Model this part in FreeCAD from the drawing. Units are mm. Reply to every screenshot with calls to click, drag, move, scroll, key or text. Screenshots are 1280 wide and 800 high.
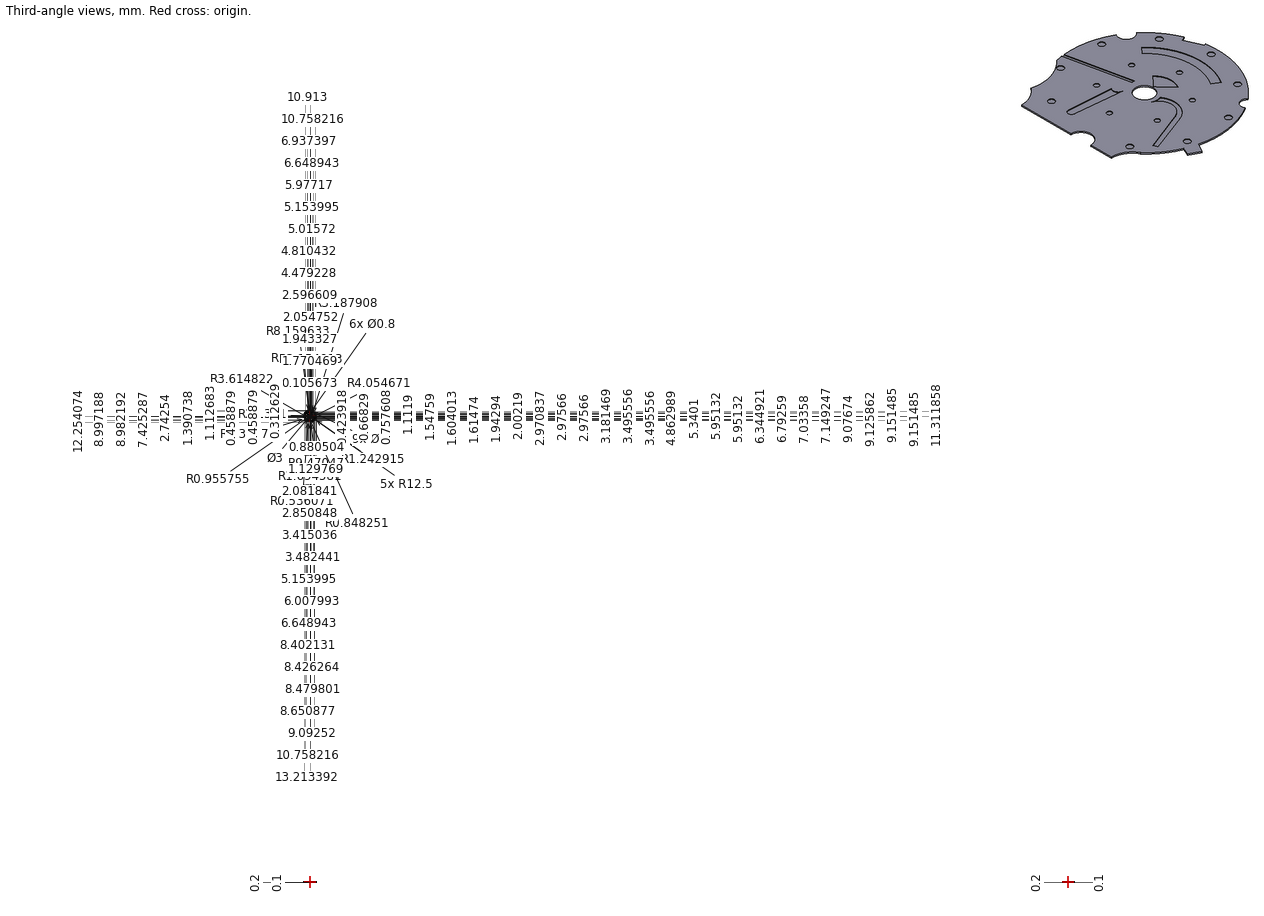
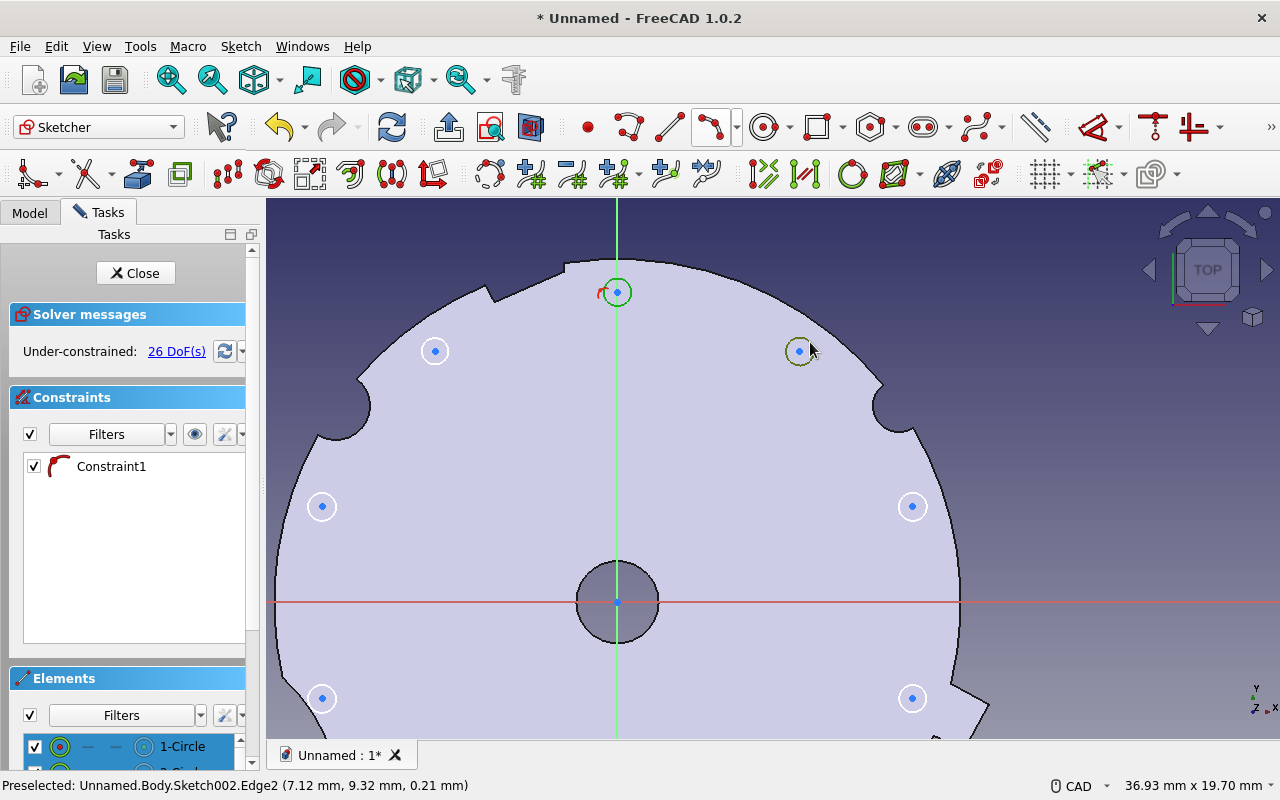
click(923, 497)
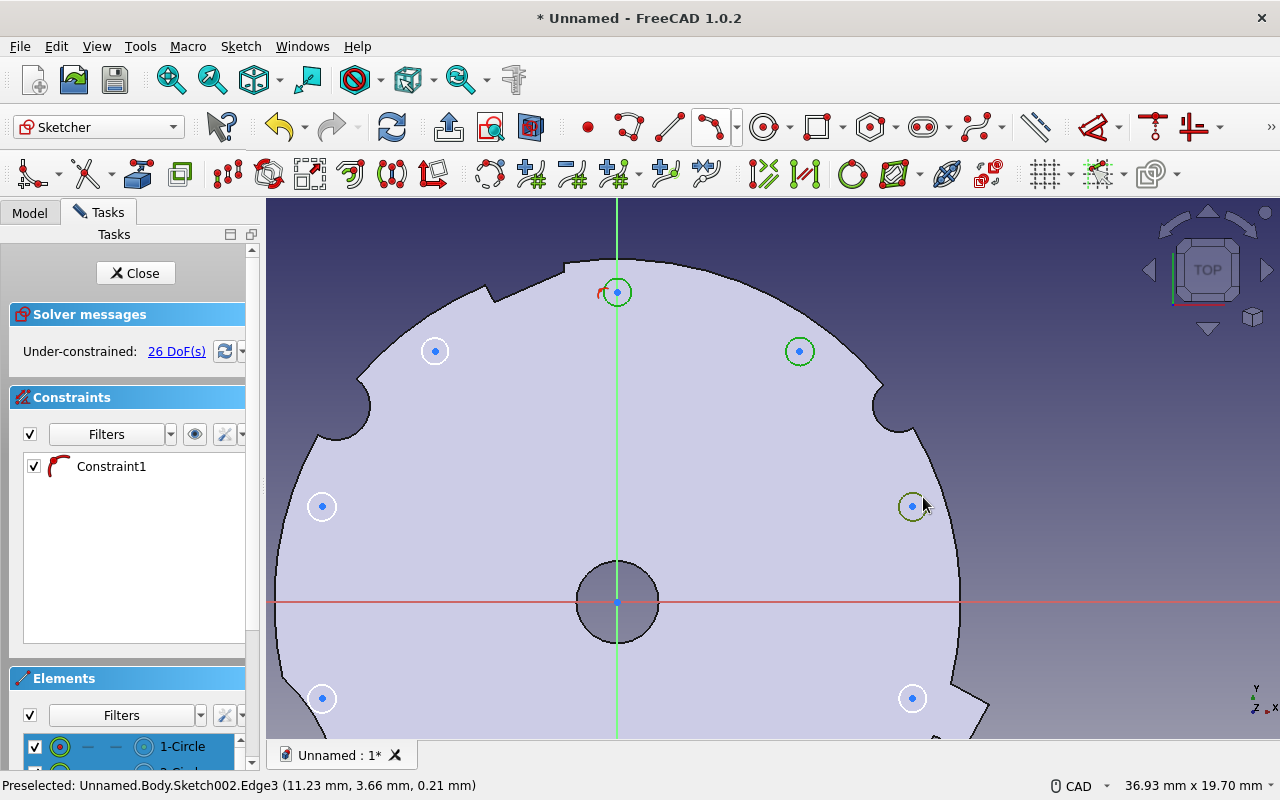
click(922, 689)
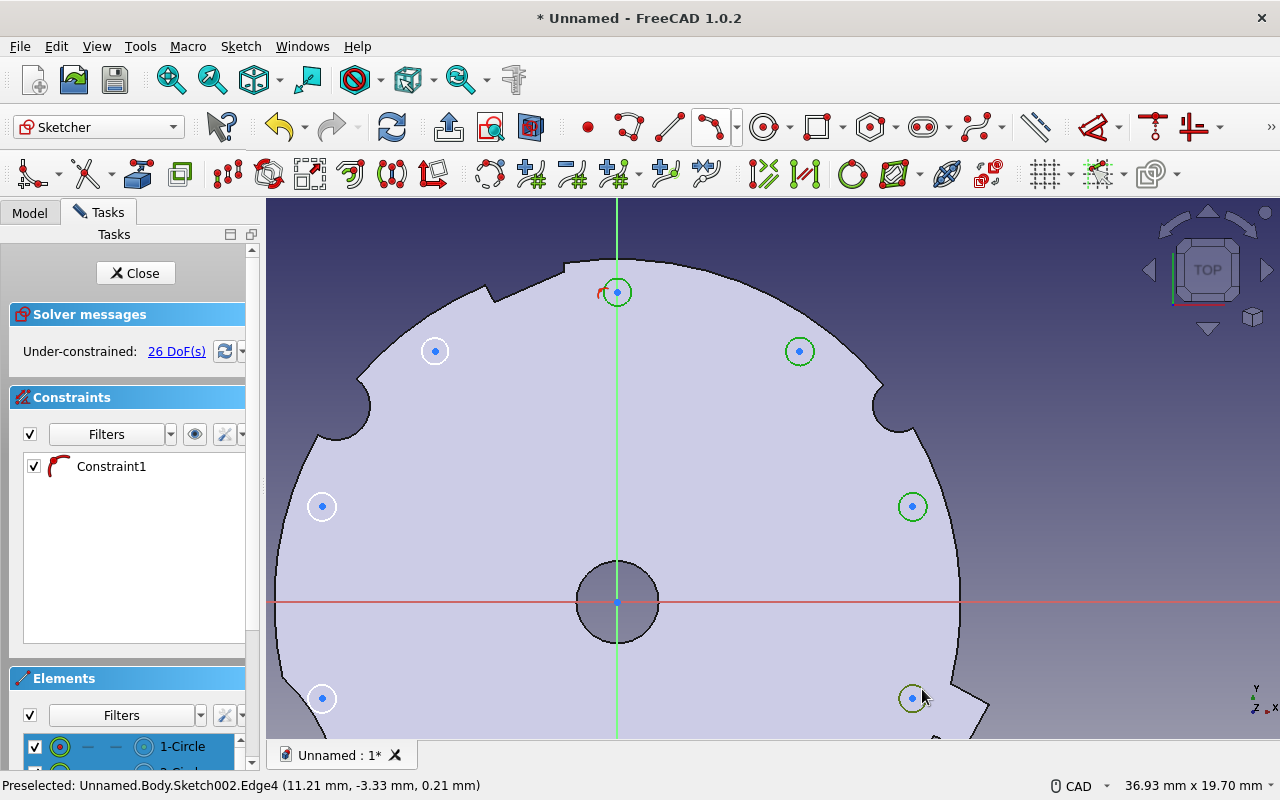
scroll(810, 342, down, 3)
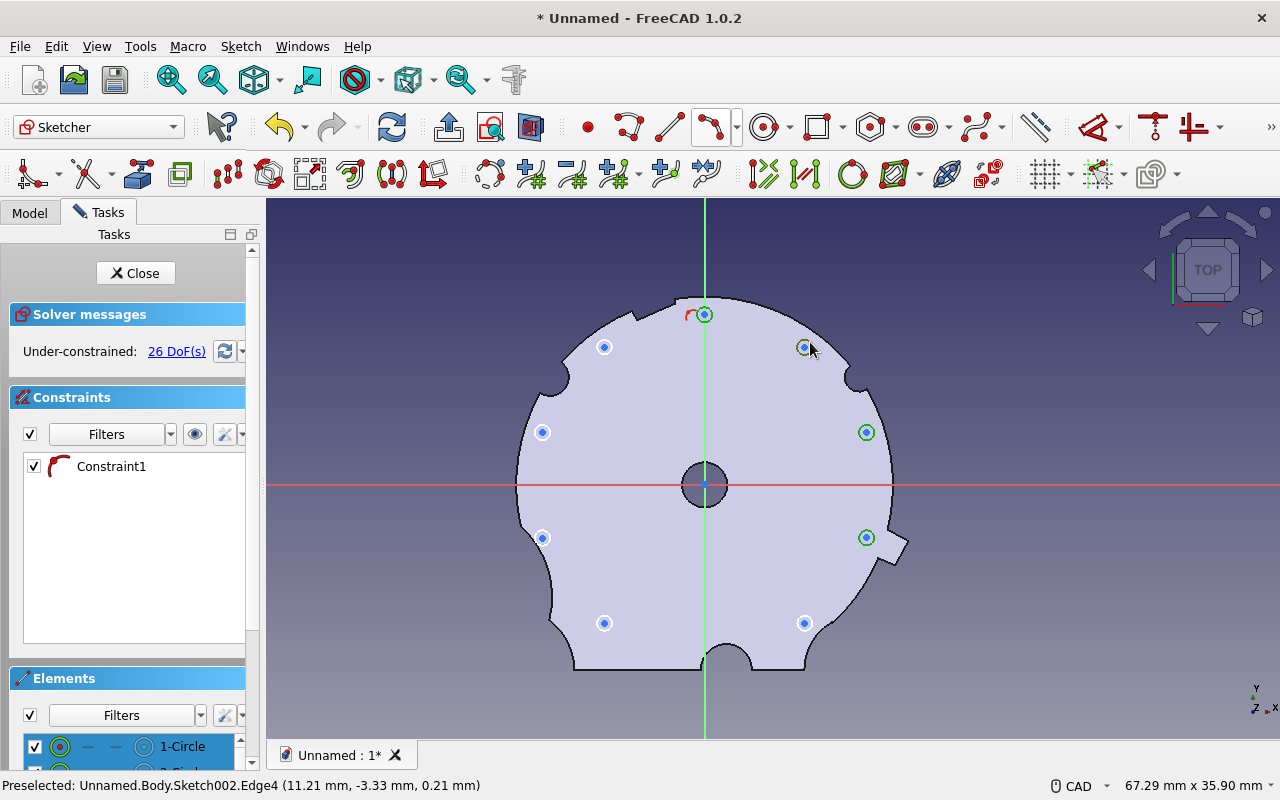
scroll(810, 618, up, 4)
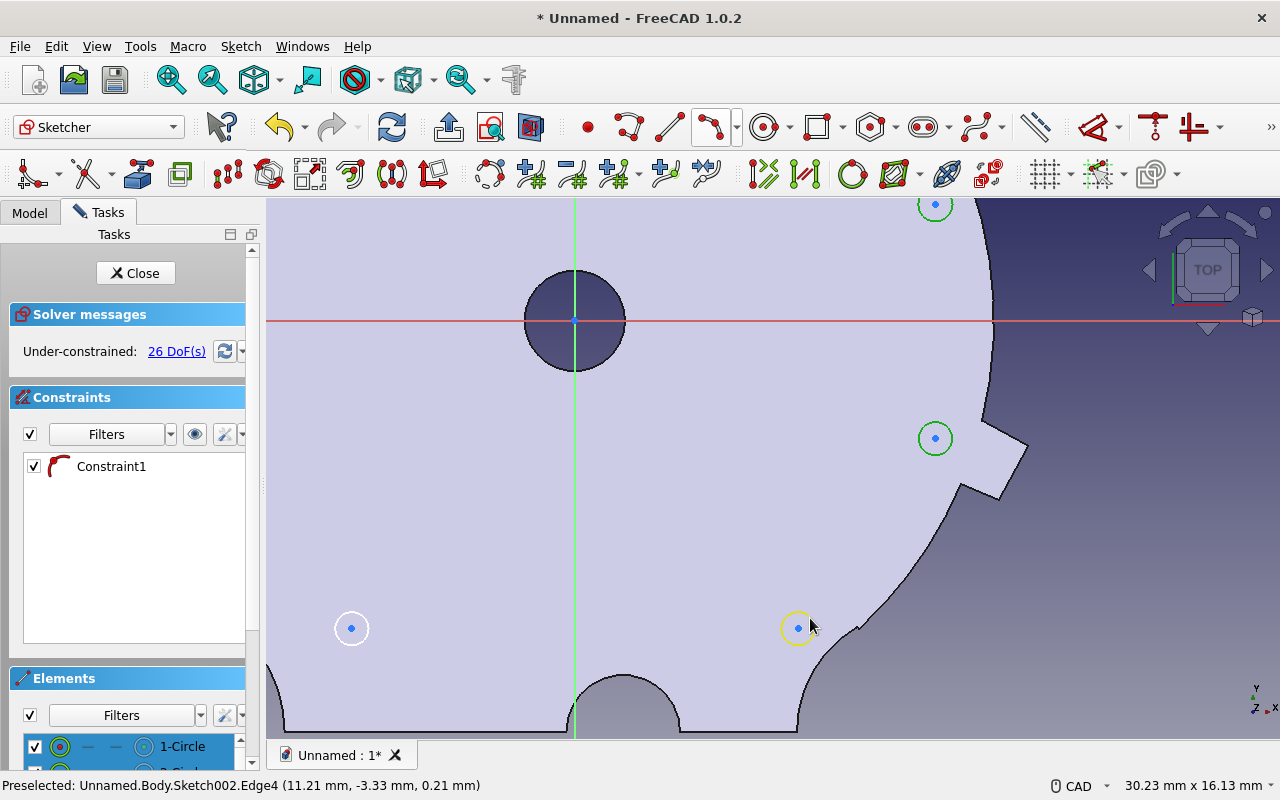
click(810, 617)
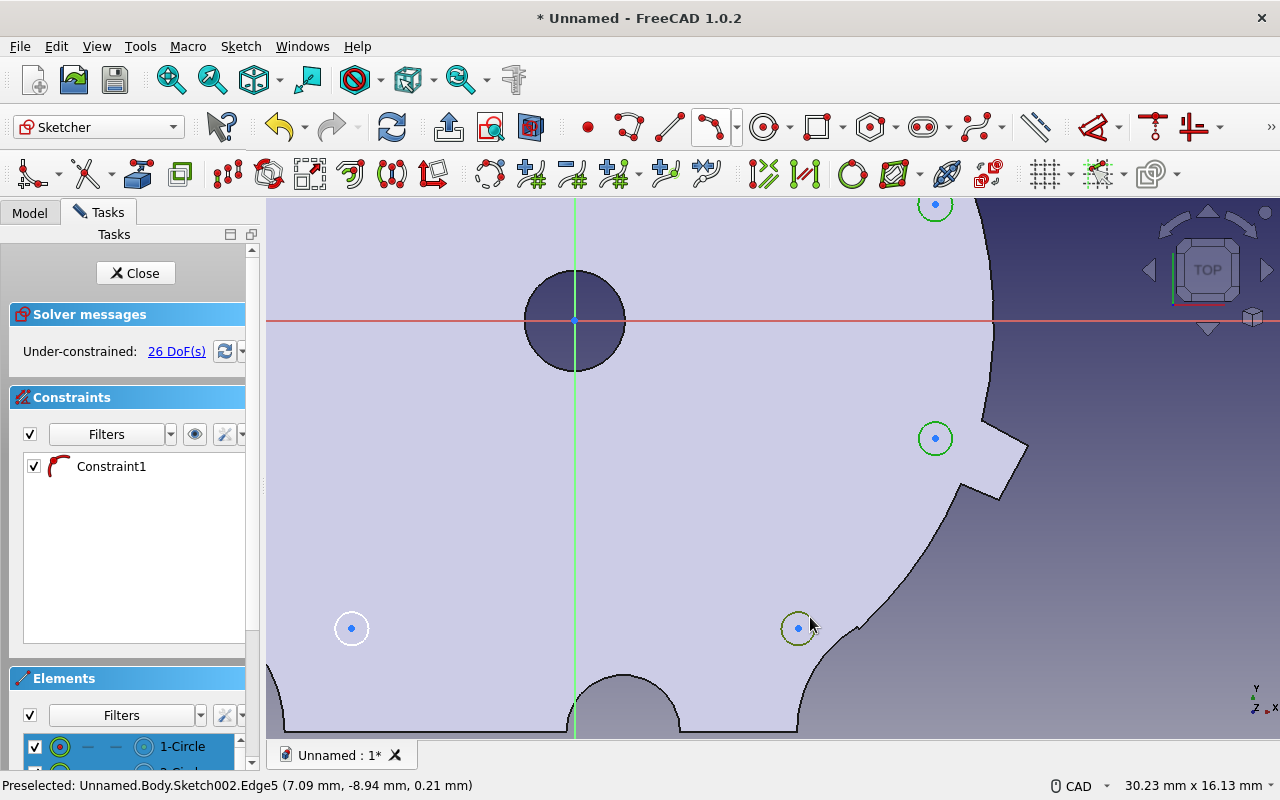
click(364, 617)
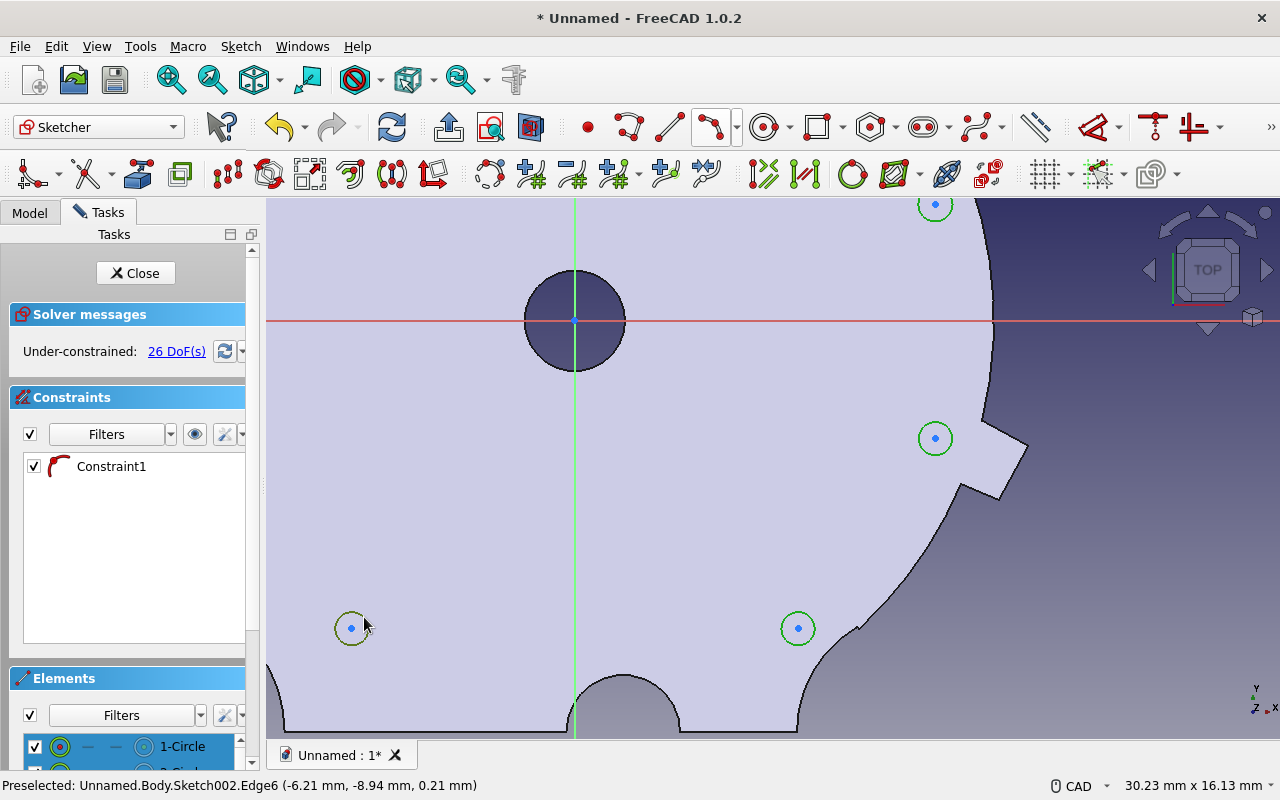
scroll(810, 619, down, 4)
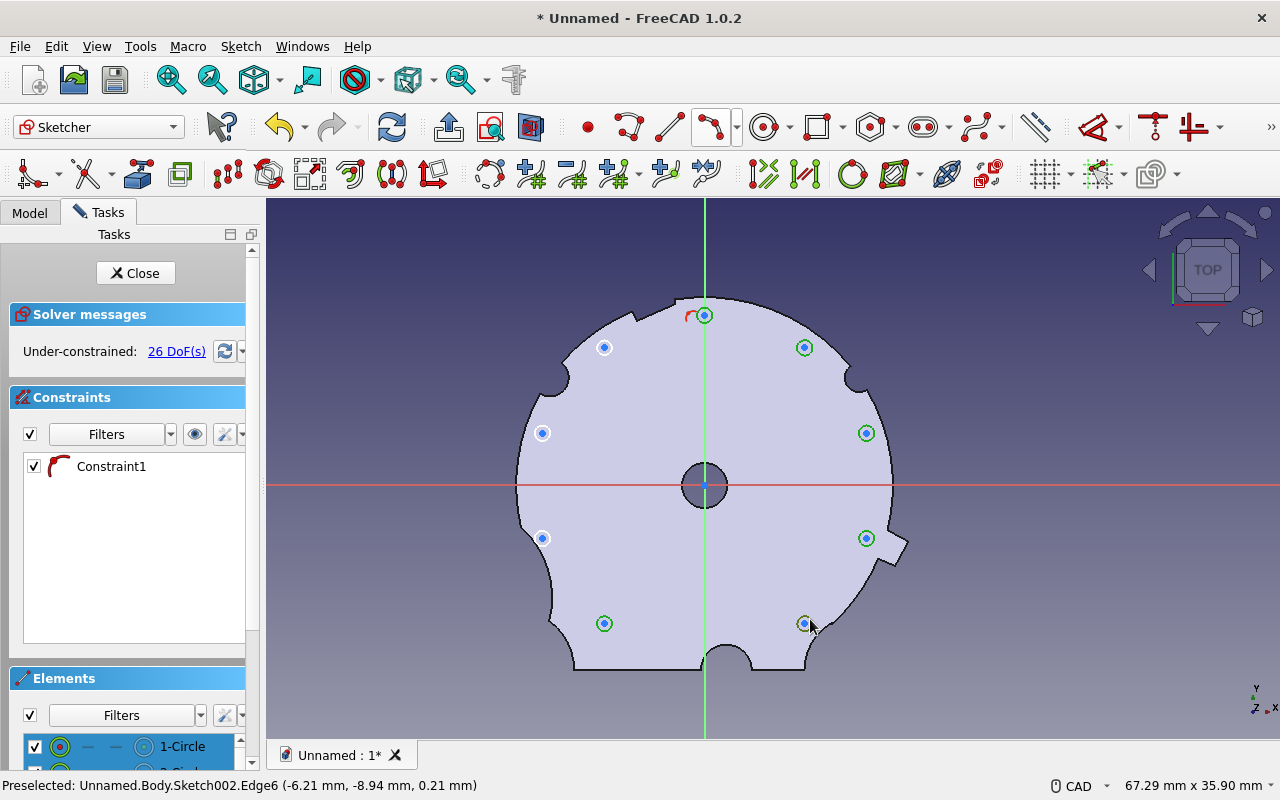
scroll(548, 533, up, 3)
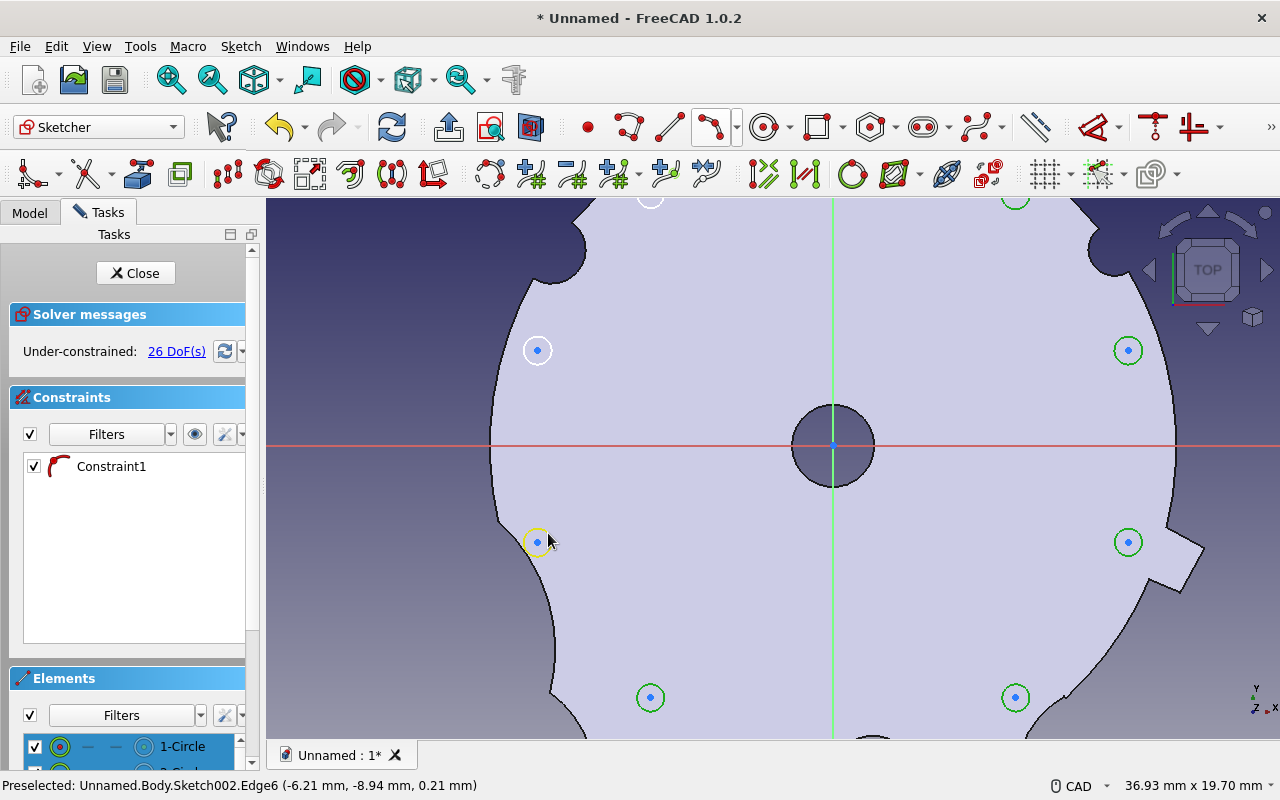
click(547, 533)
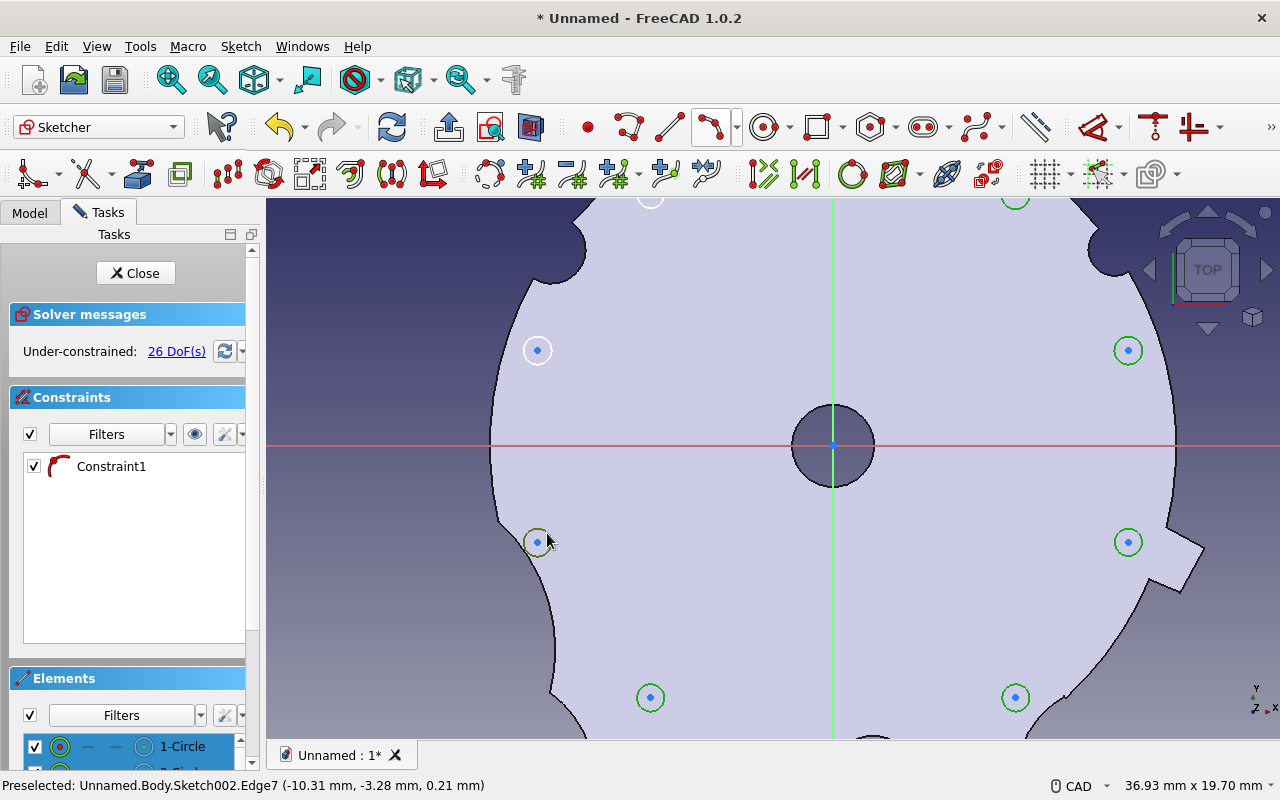
click(547, 341)